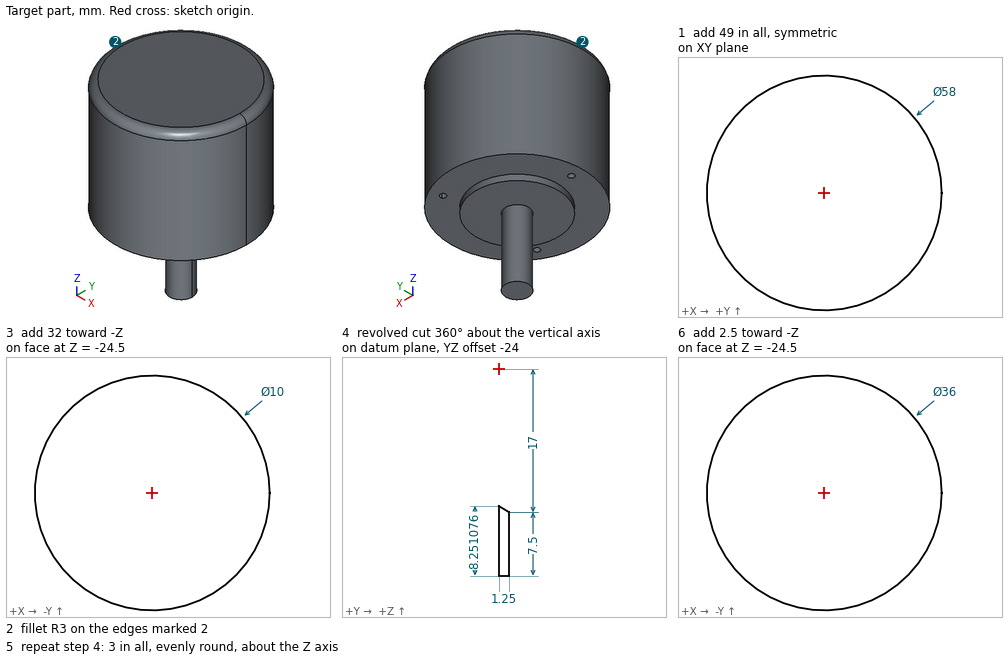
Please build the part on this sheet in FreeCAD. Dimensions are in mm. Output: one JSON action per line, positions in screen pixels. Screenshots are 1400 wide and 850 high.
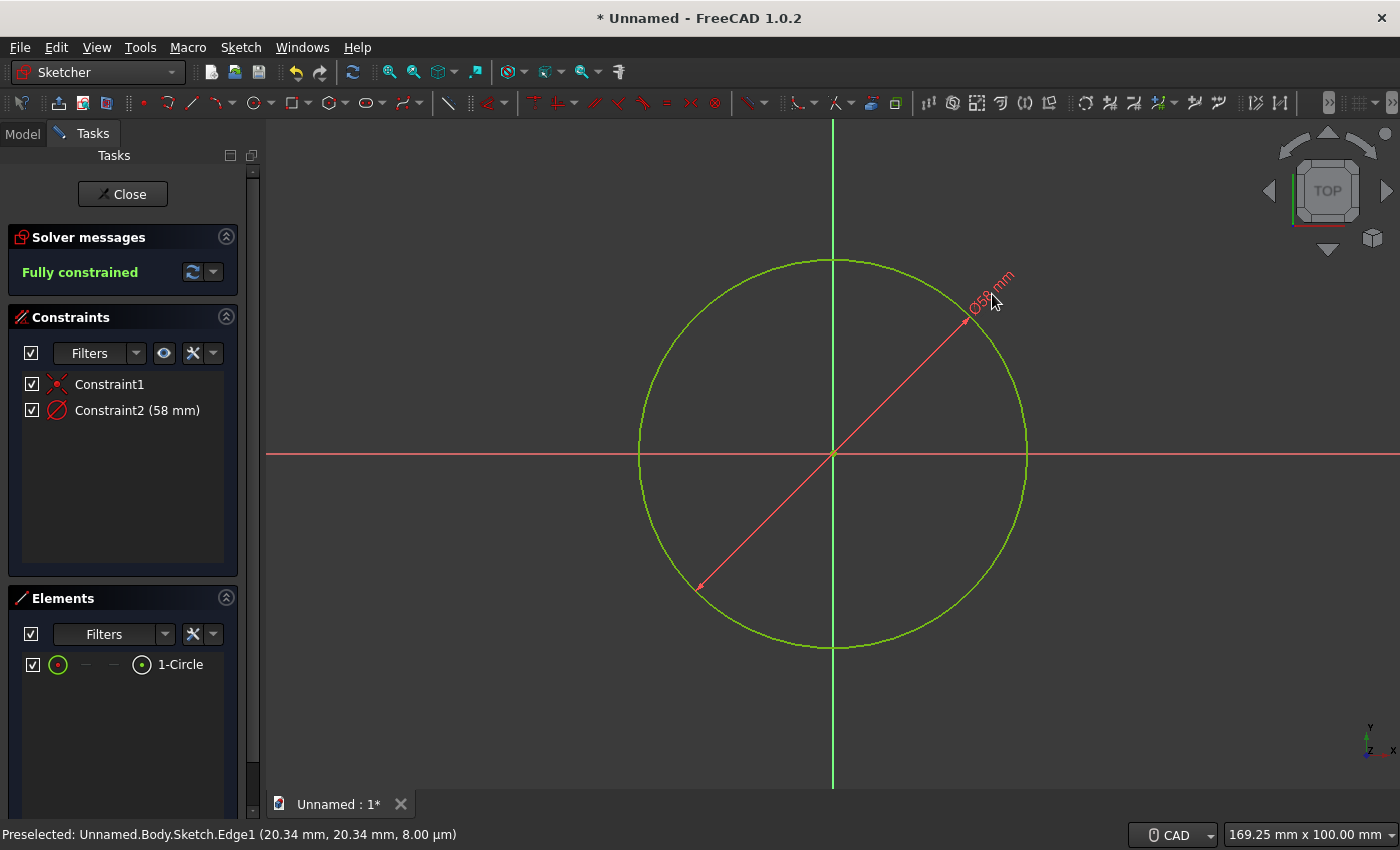
{"action": "left_click", "coordinate": [123, 194]}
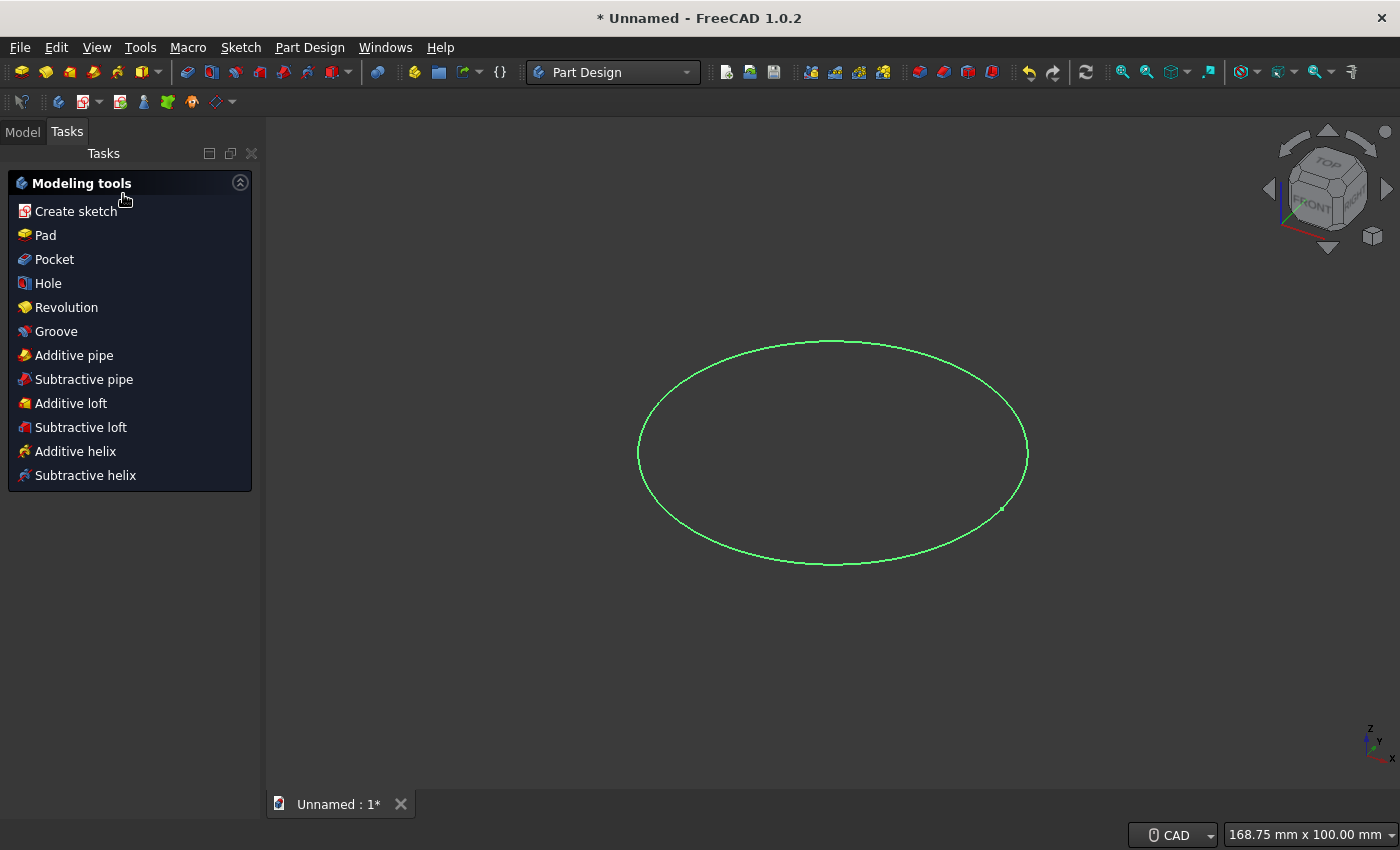
{"action": "left_click", "coordinate": [22, 72]}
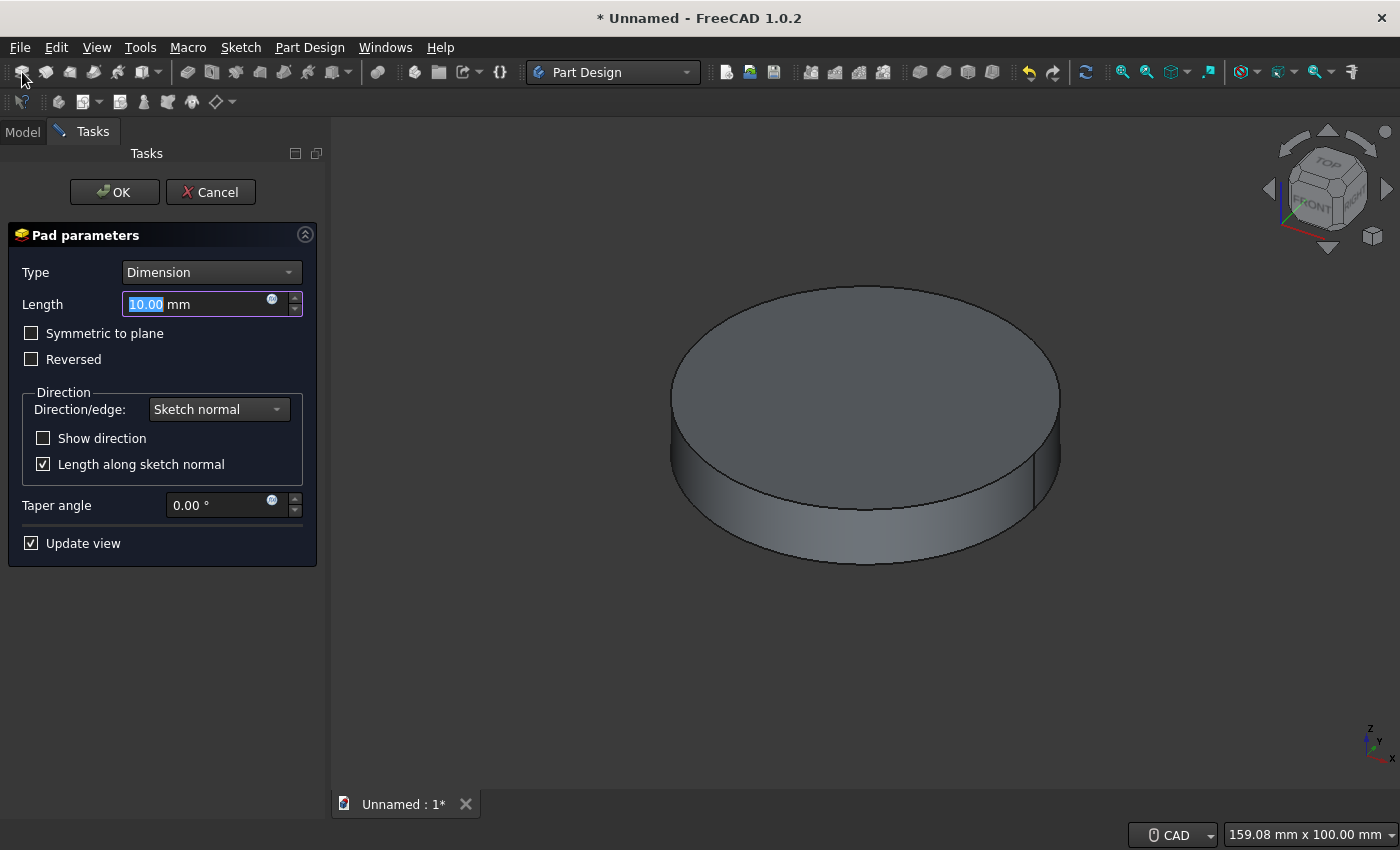
{"action": "type", "text": "49"}
{"action": "key", "text": "Tab"}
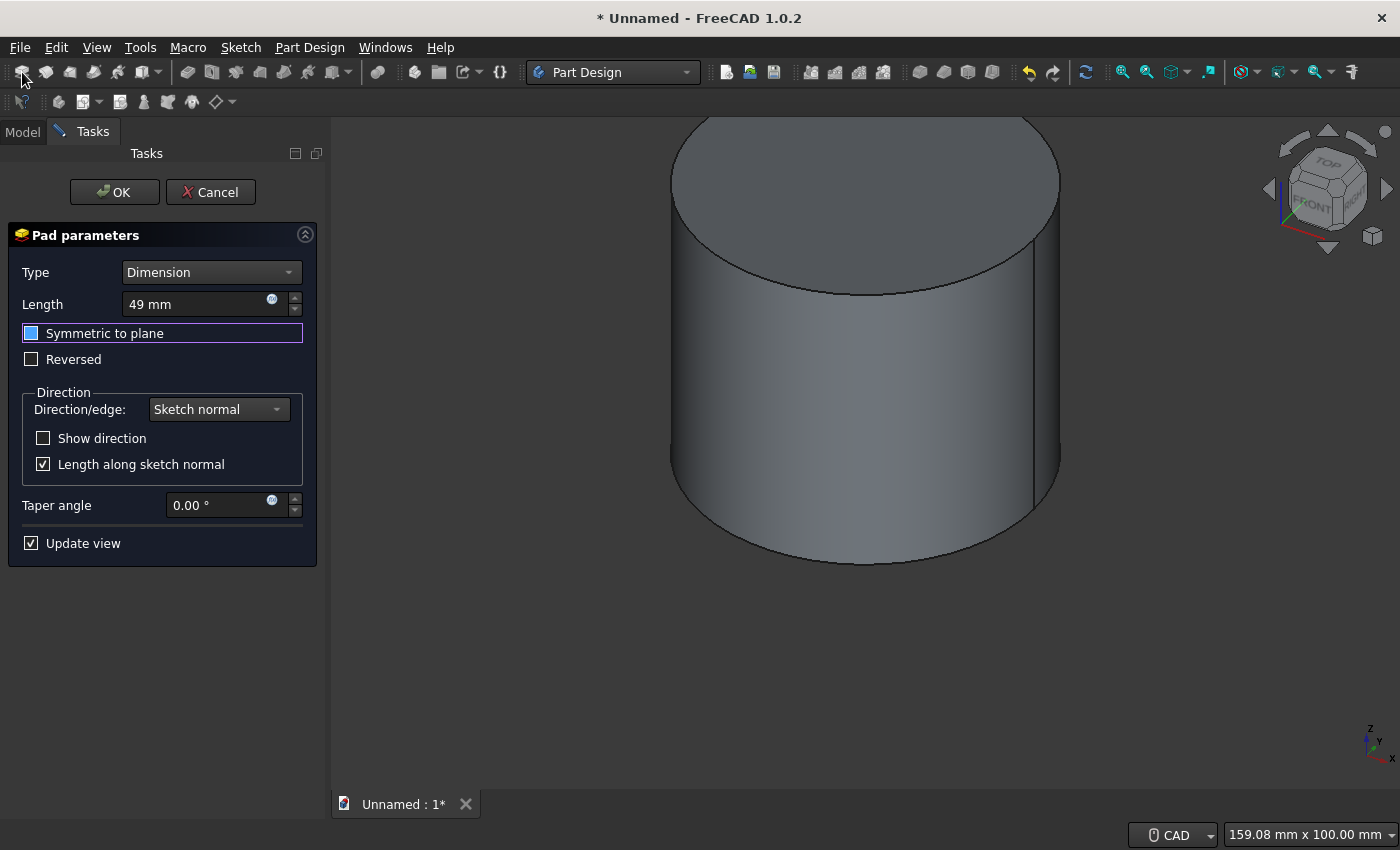
{"action": "left_click", "coordinate": [30, 333]}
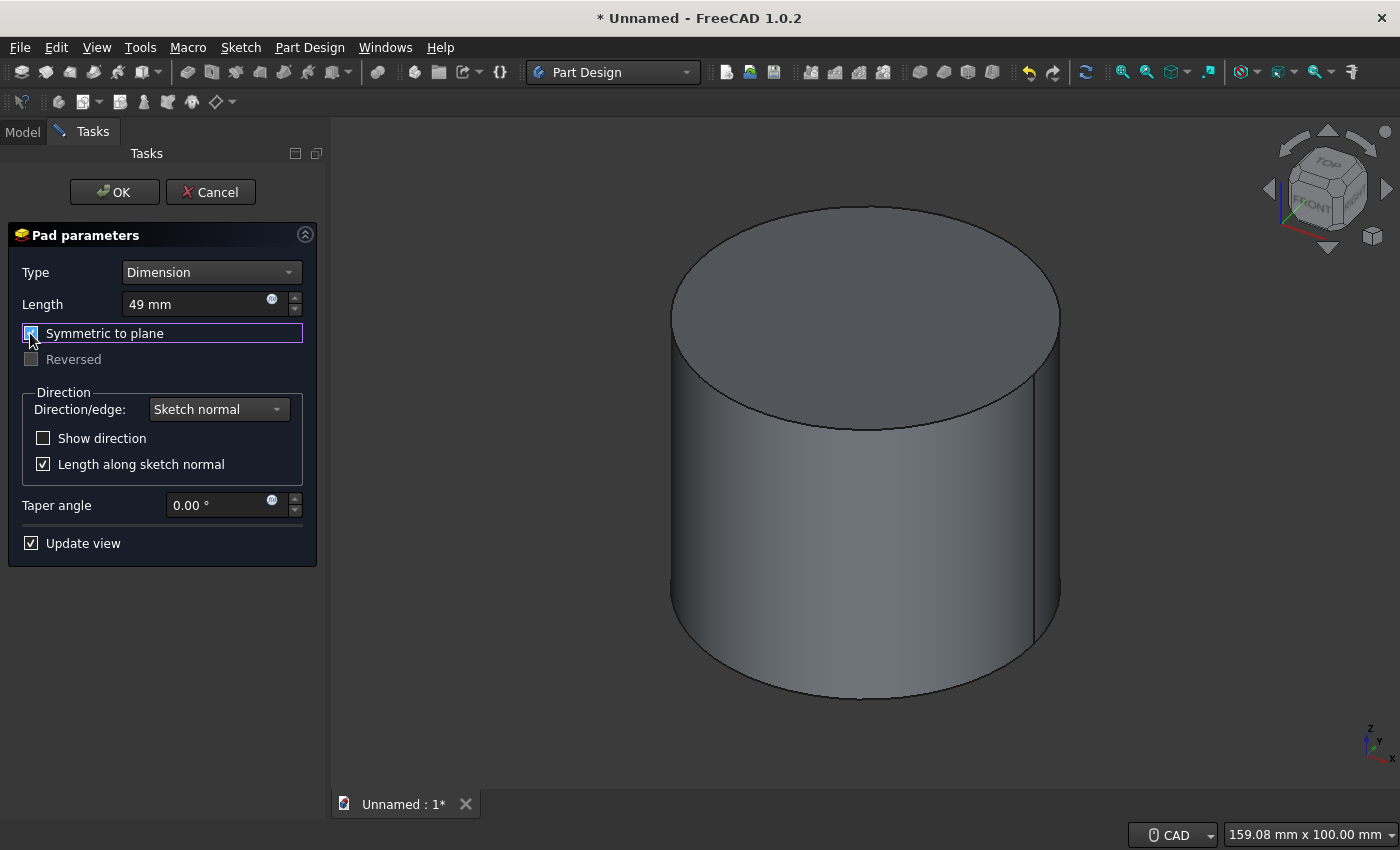
{"action": "left_click", "coordinate": [115, 192]}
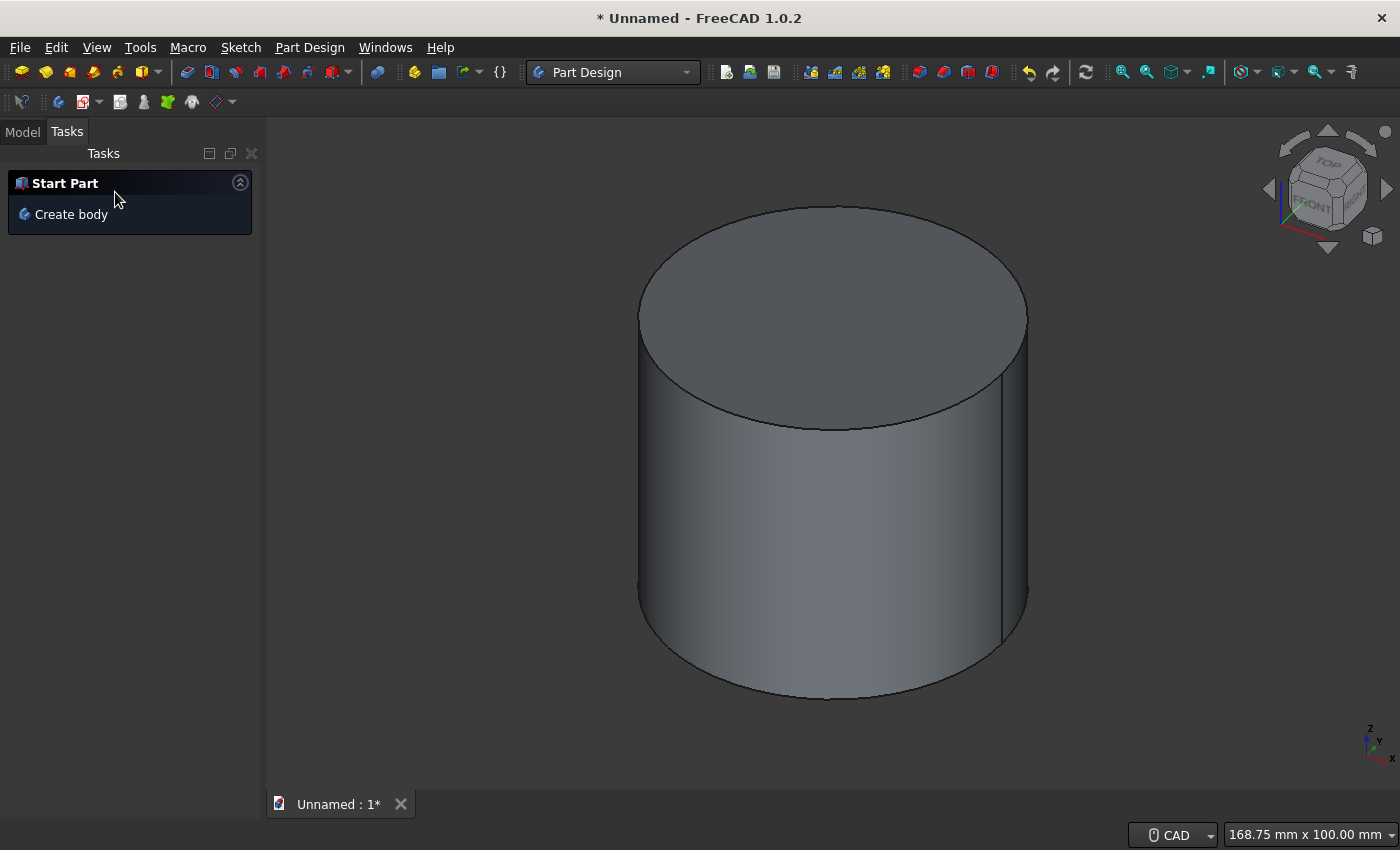
{"action": "left_click", "coordinate": [639, 329]}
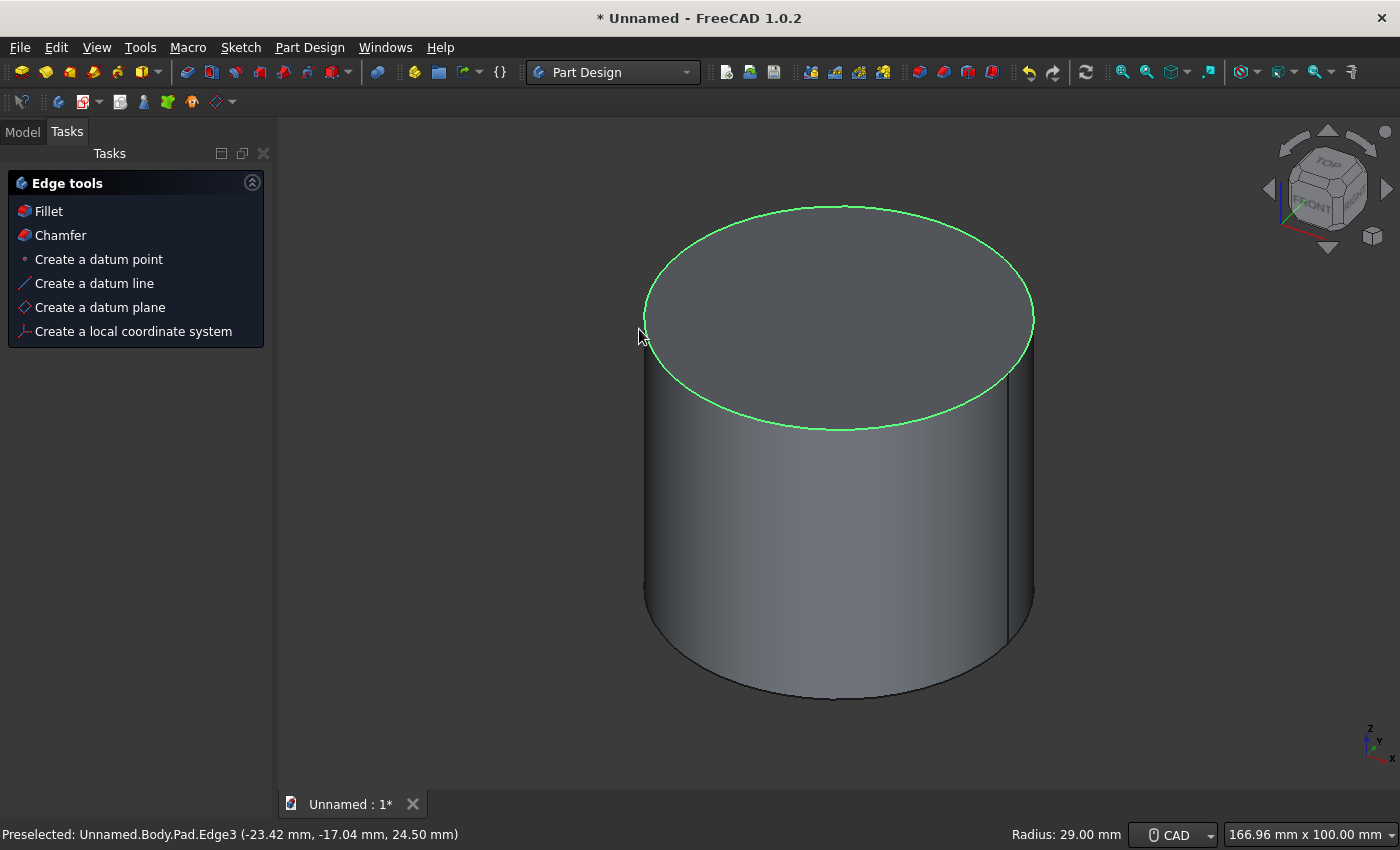
{"action": "left_click", "coordinate": [920, 72]}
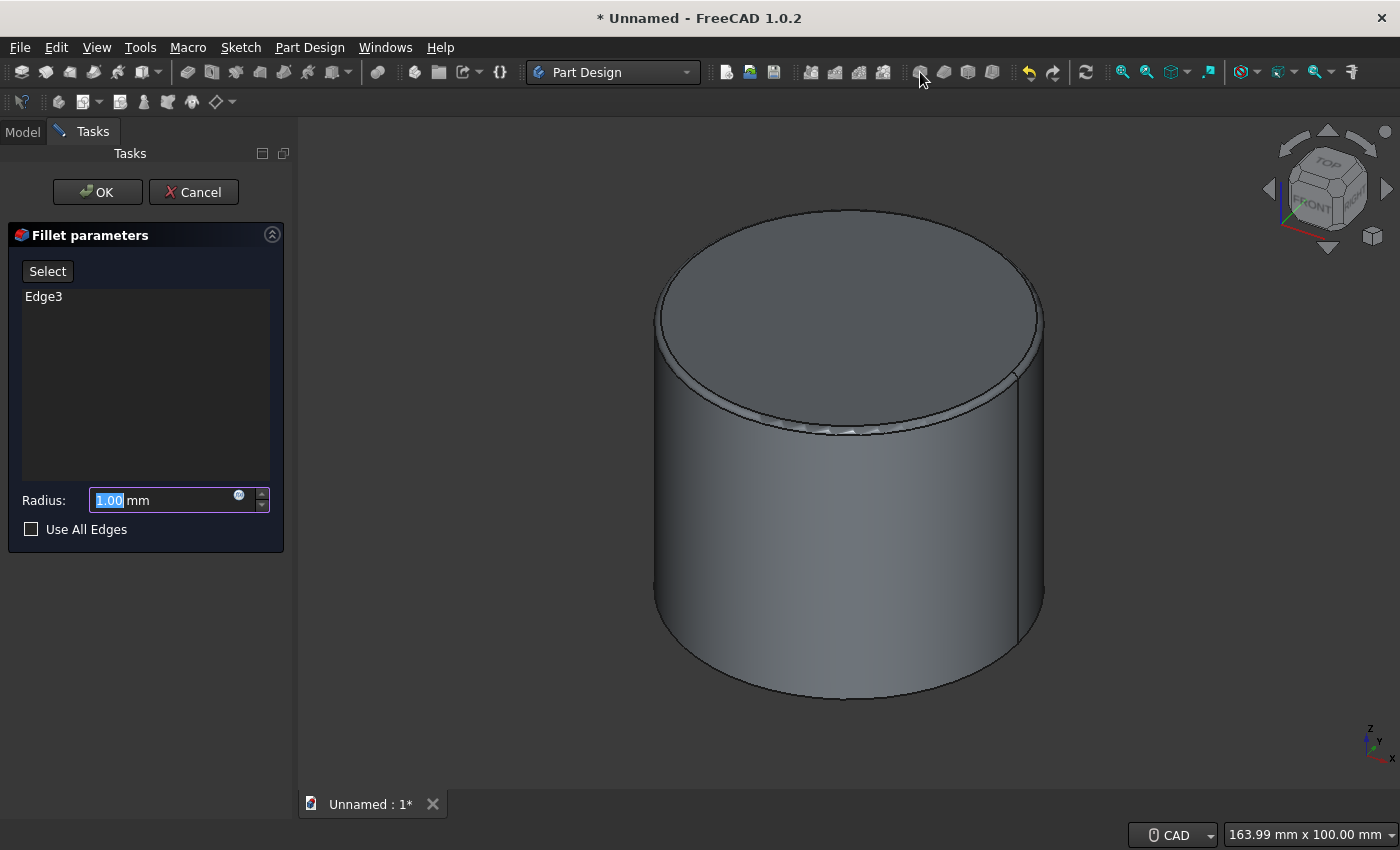
{"action": "type", "text": "3"}
{"action": "key", "text": "Tab"}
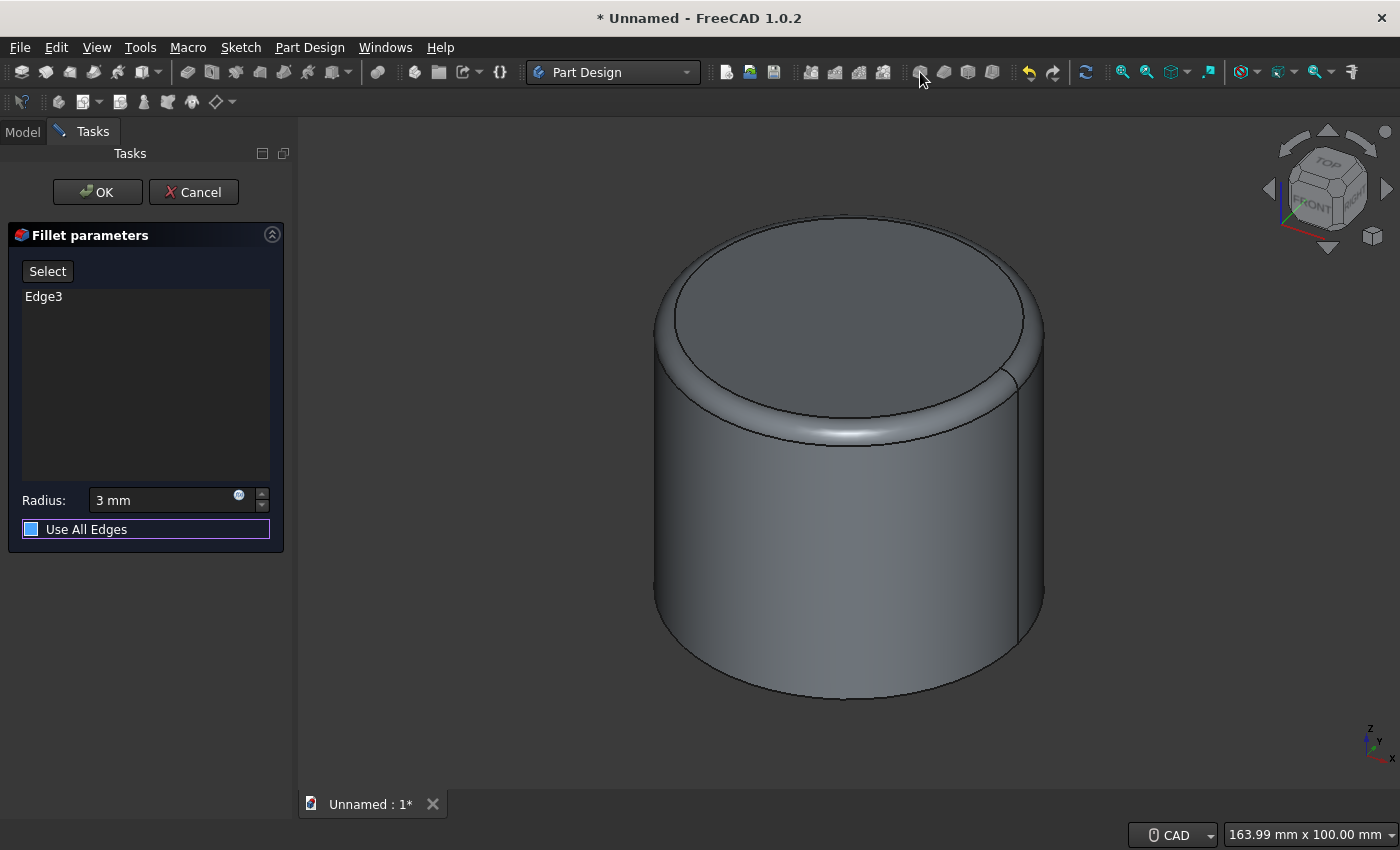
{"action": "left_click", "coordinate": [98, 192]}